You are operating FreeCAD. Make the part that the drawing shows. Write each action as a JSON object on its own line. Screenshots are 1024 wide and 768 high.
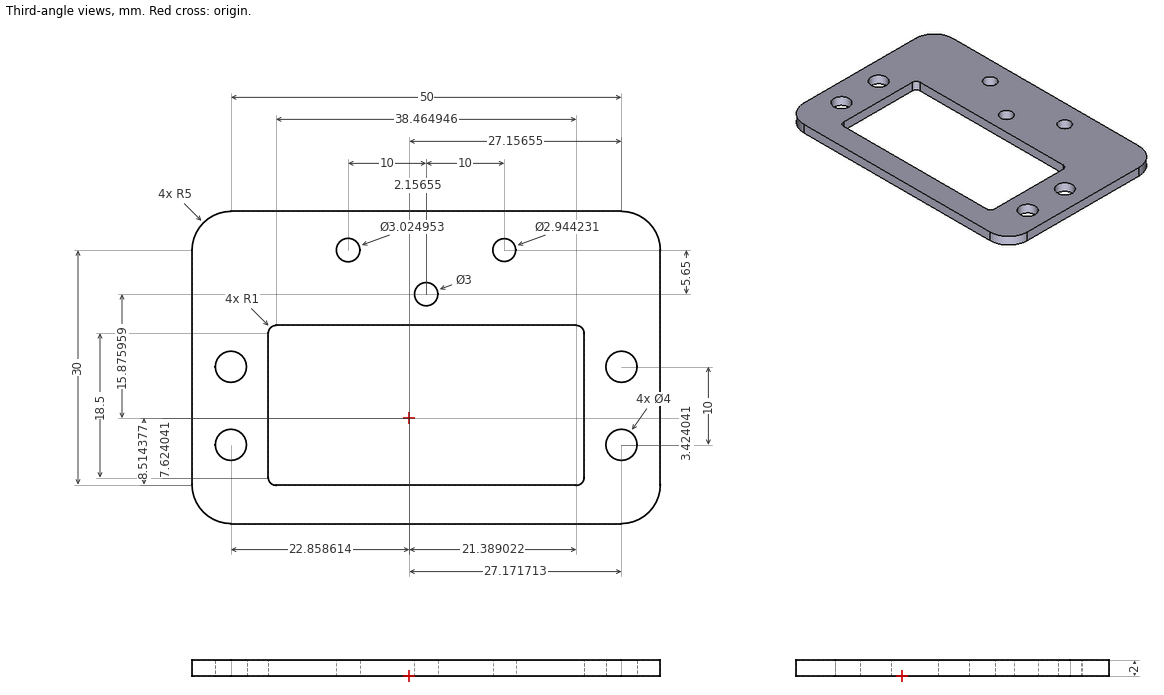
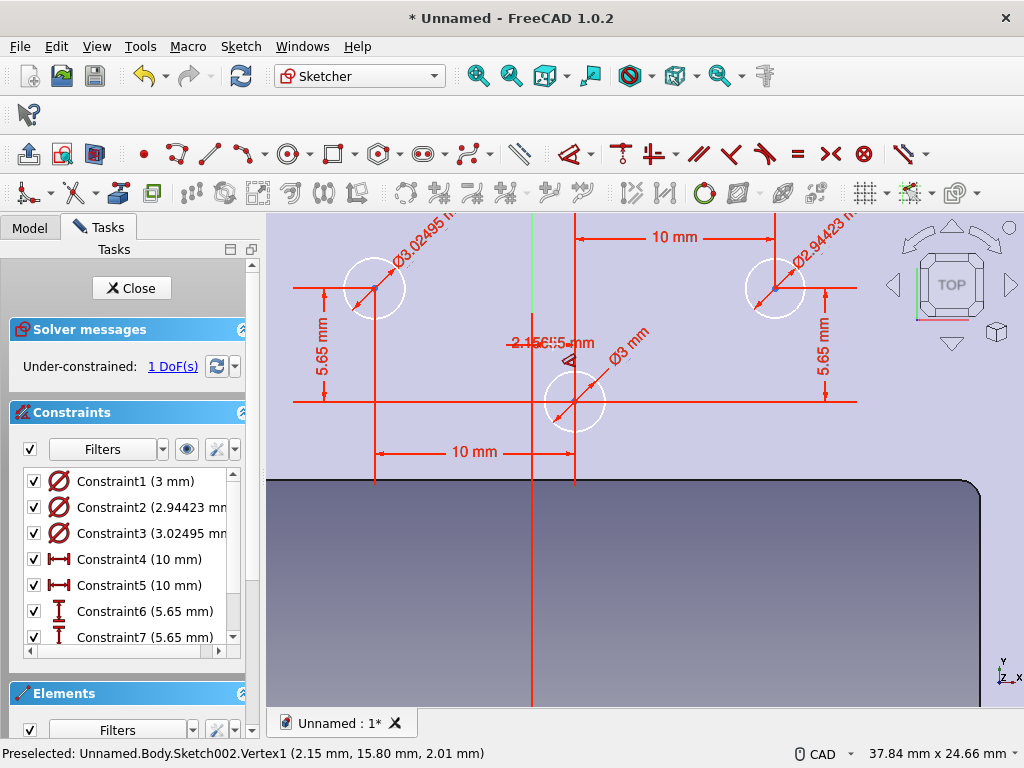
{"action": "left_click", "coordinate": [575, 402]}
{"action": "left_click", "coordinate": [498, 540]}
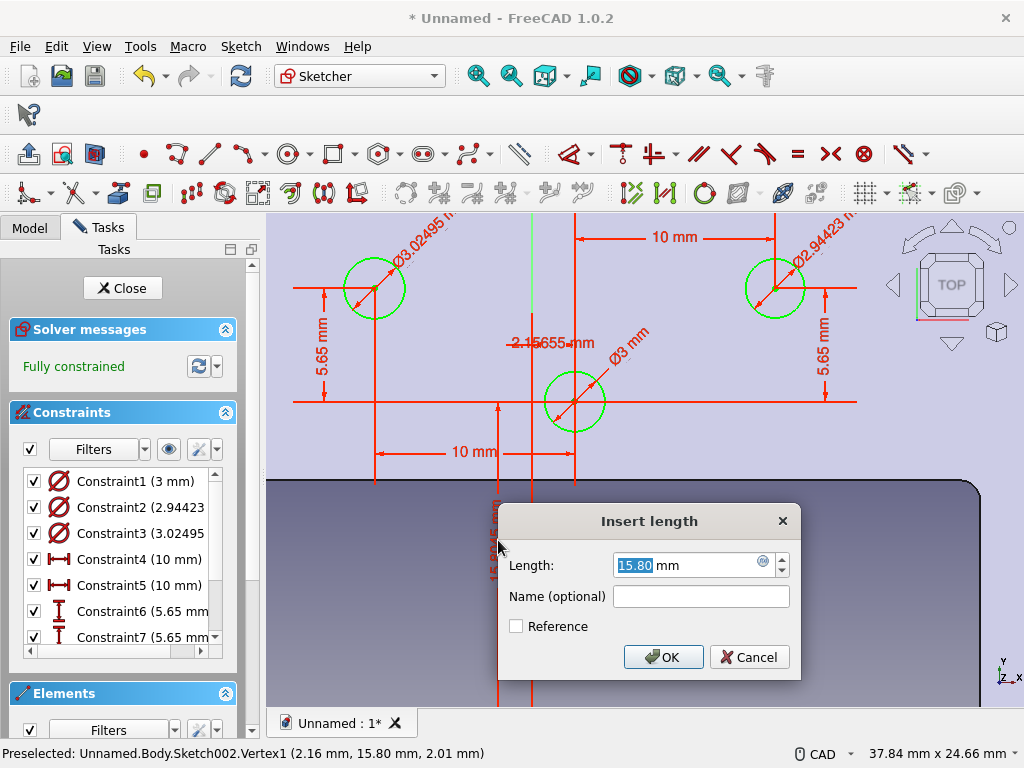
{"action": "type", "text": "15.875959"}
{"action": "key", "text": "Return"}
{"action": "key", "text": "Escape"}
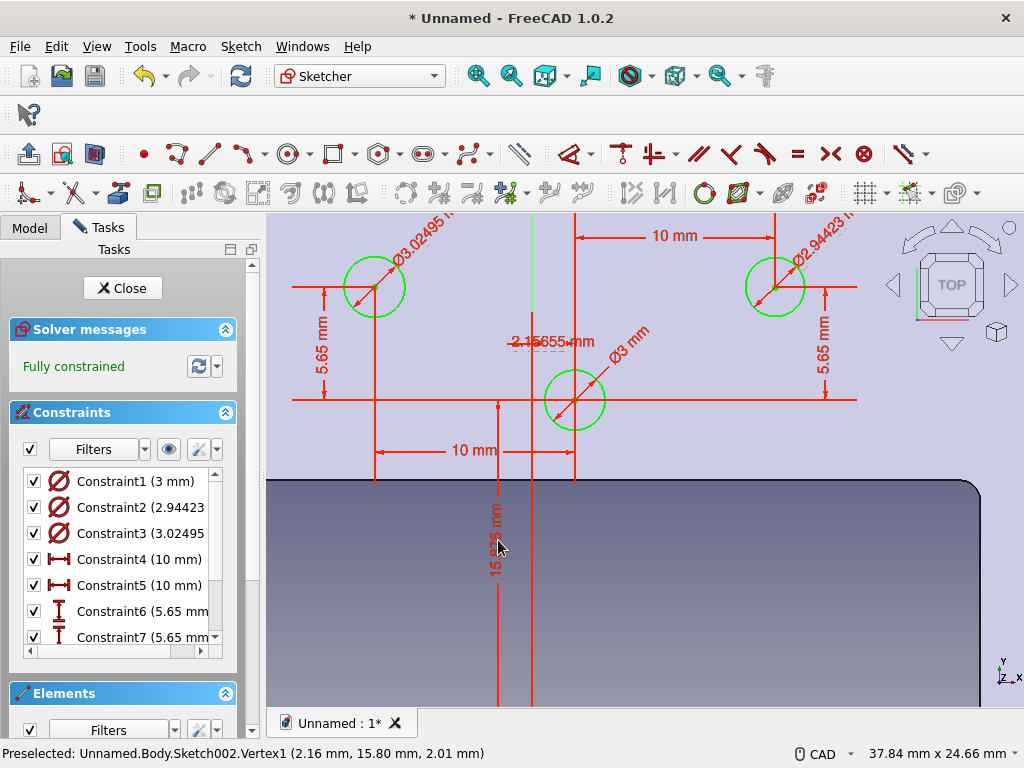
{"action": "left_click", "coordinate": [123, 288]}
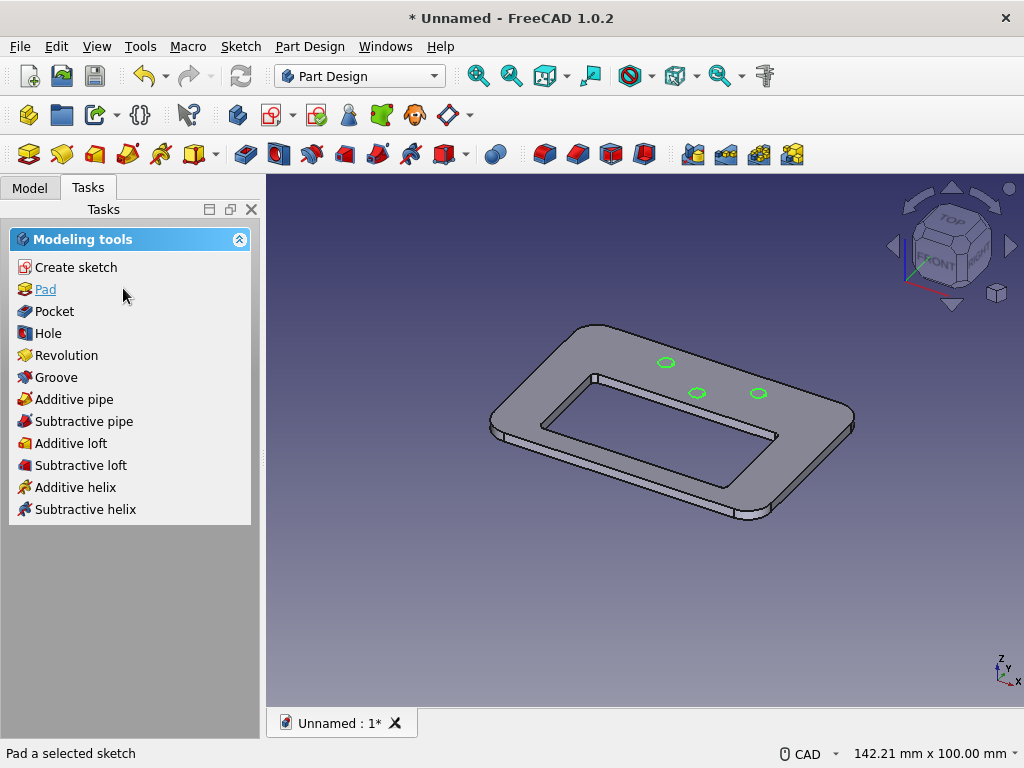
{"action": "left_click", "coordinate": [246, 154]}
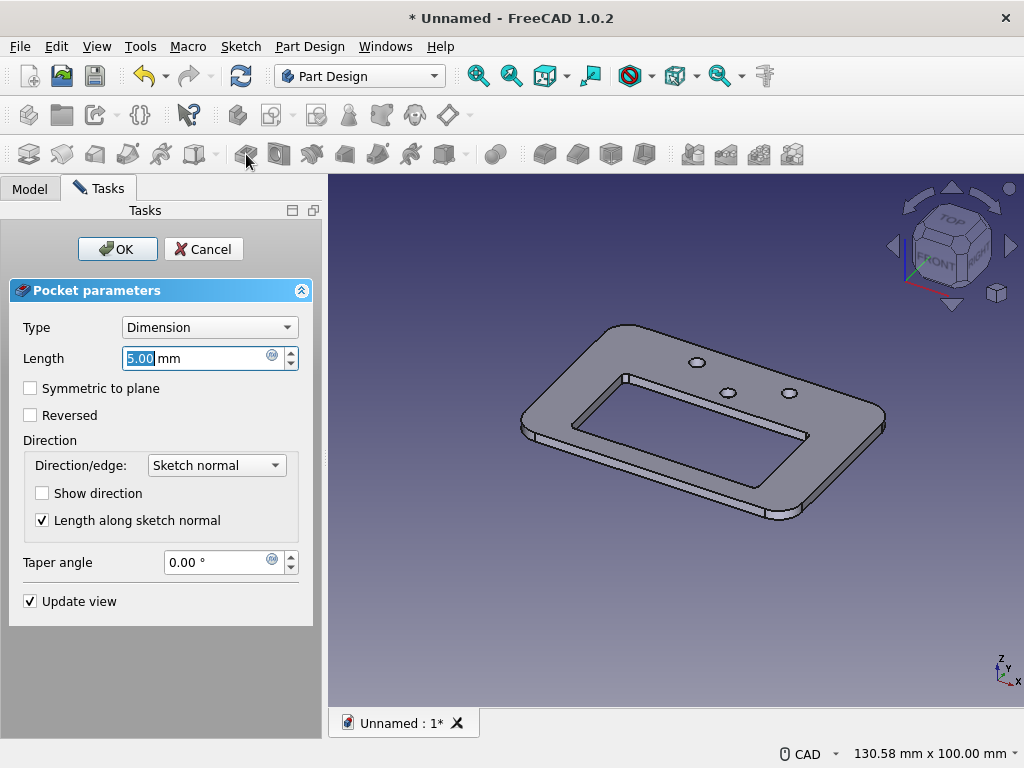
{"action": "left_click", "coordinate": [210, 328]}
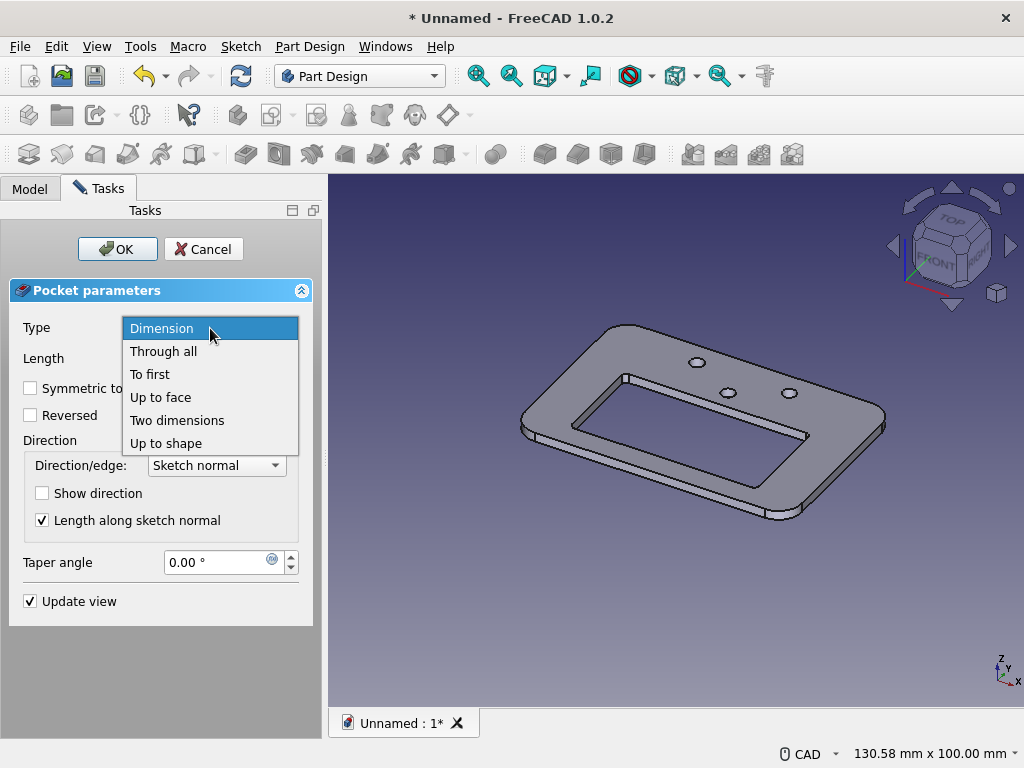
{"action": "left_click", "coordinate": [208, 352]}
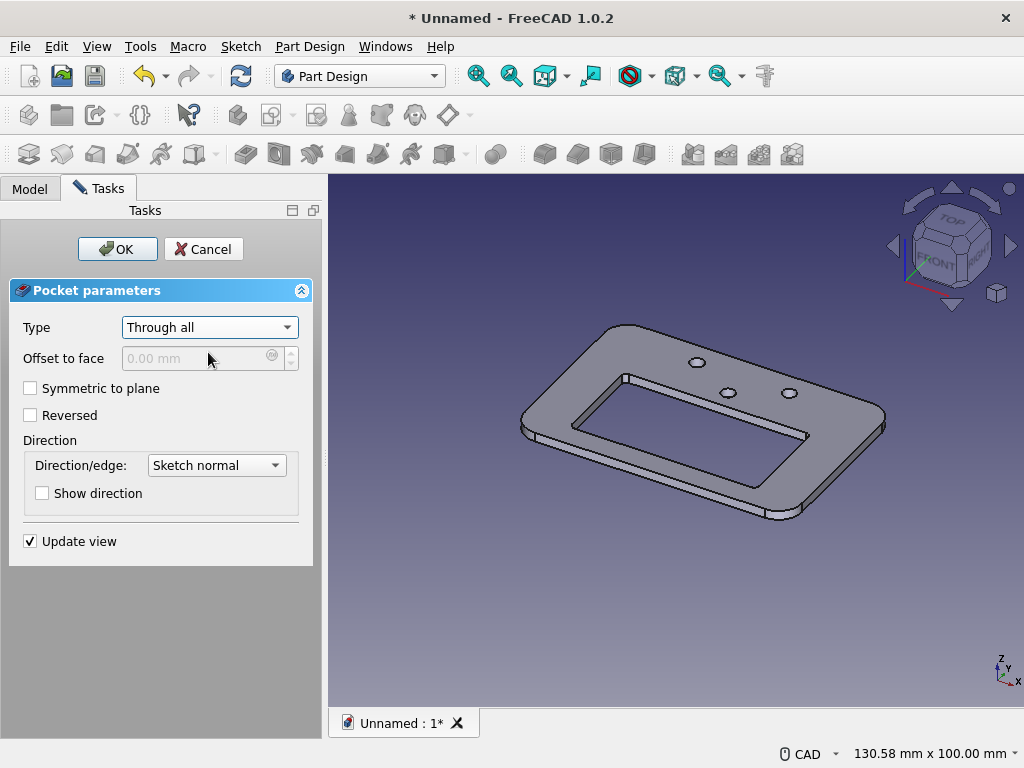
{"action": "left_click", "coordinate": [118, 249]}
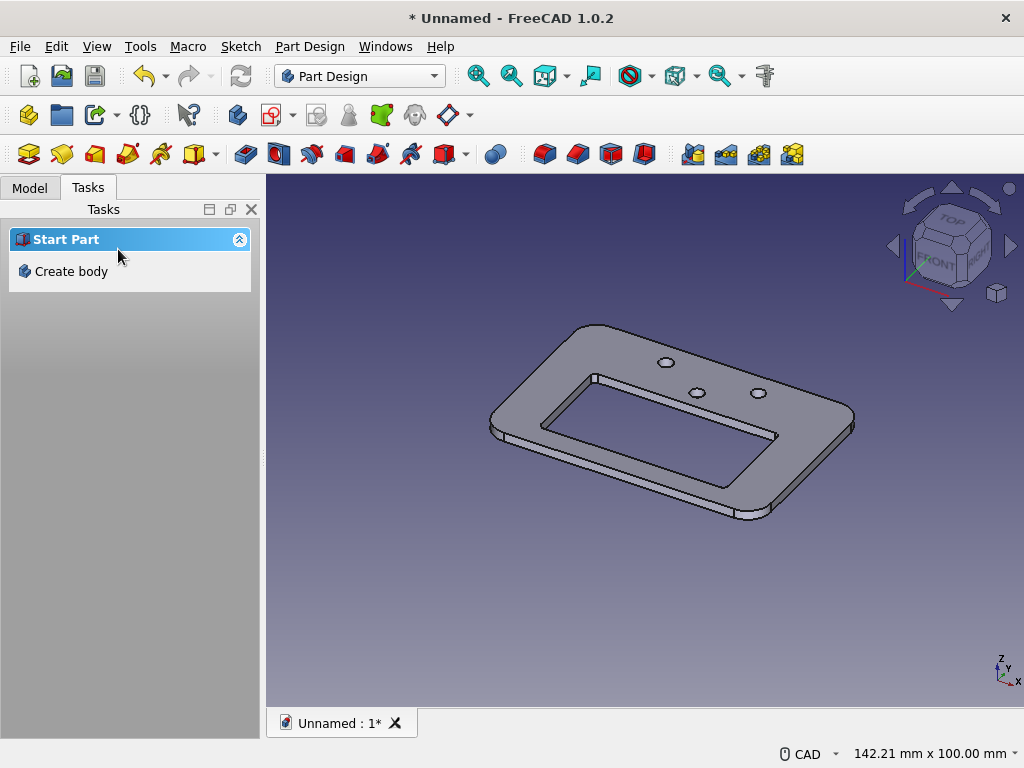
{"action": "left_click", "coordinate": [782, 413]}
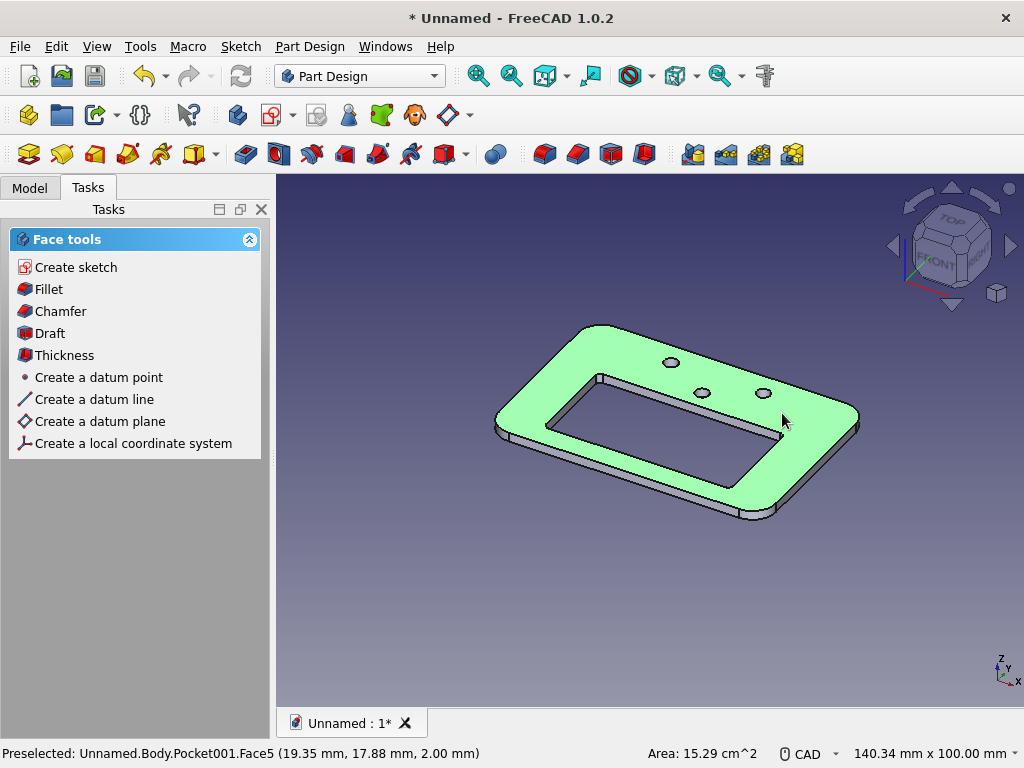
{"action": "left_click", "coordinate": [270, 116]}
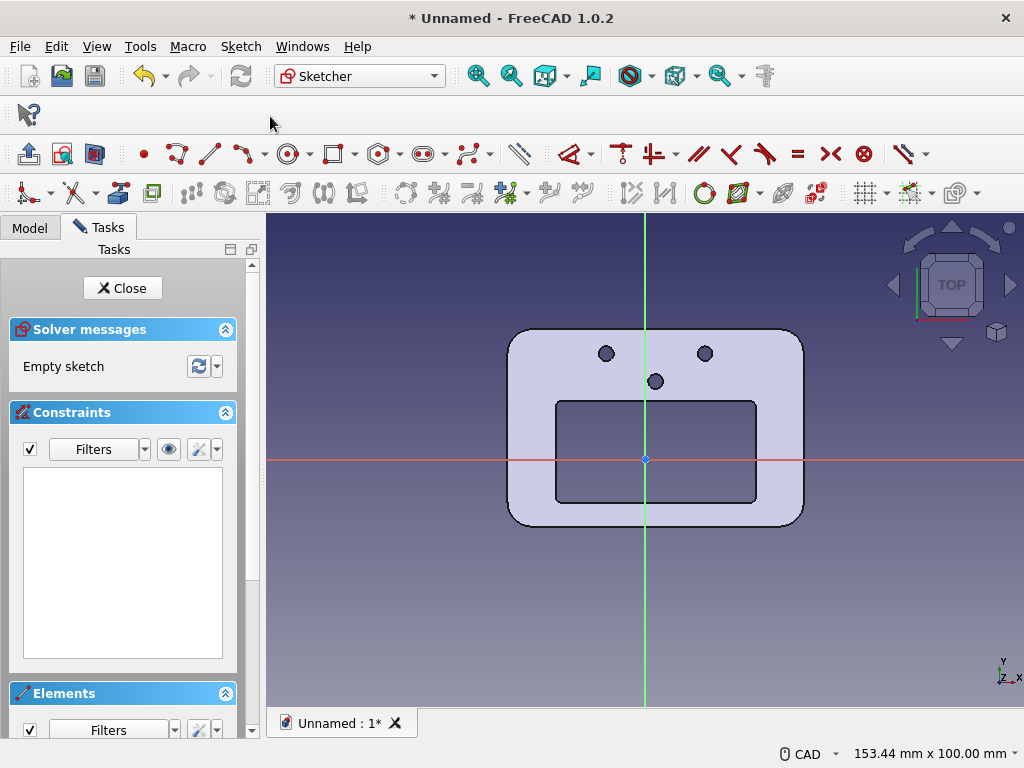
{"action": "scroll", "coordinate": [817, 436], "scroll_direction": "up", "scroll_amount": 2}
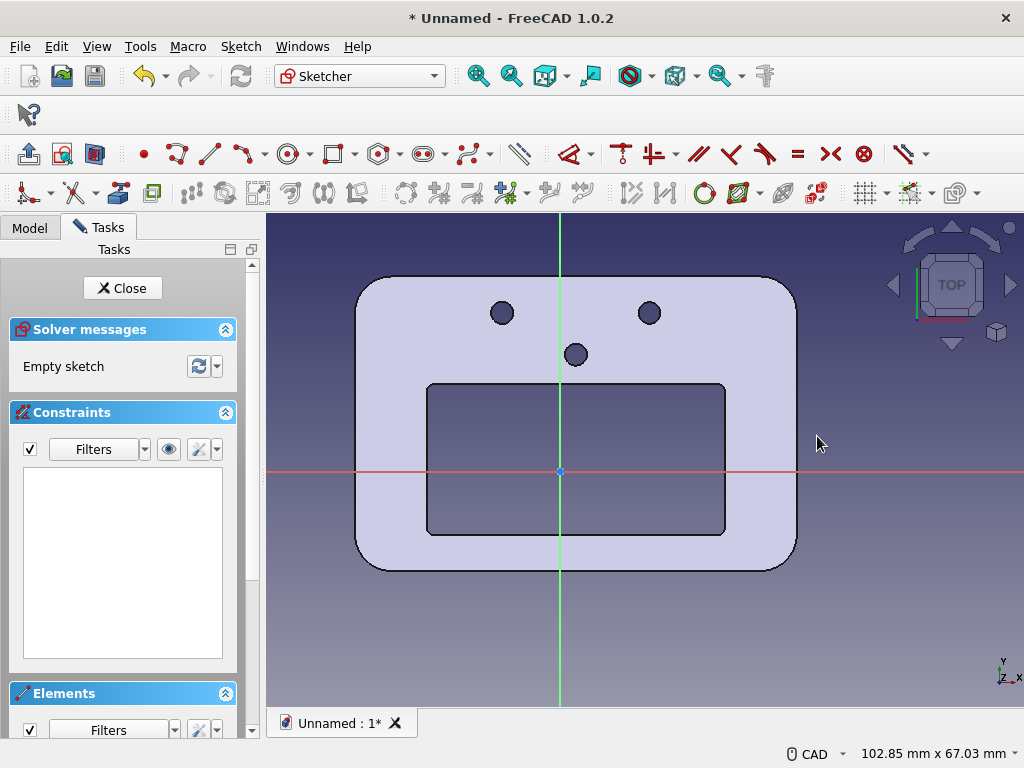
{"action": "left_click", "coordinate": [288, 154]}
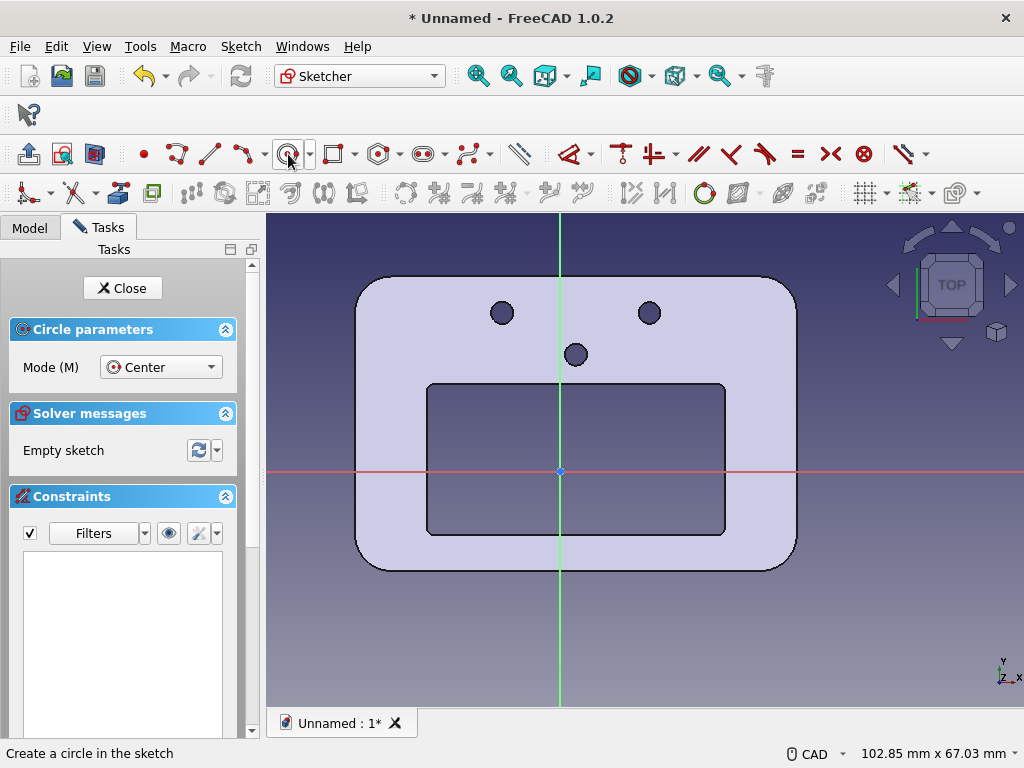
{"action": "scroll", "coordinate": [760, 497], "scroll_direction": "up", "scroll_amount": 3}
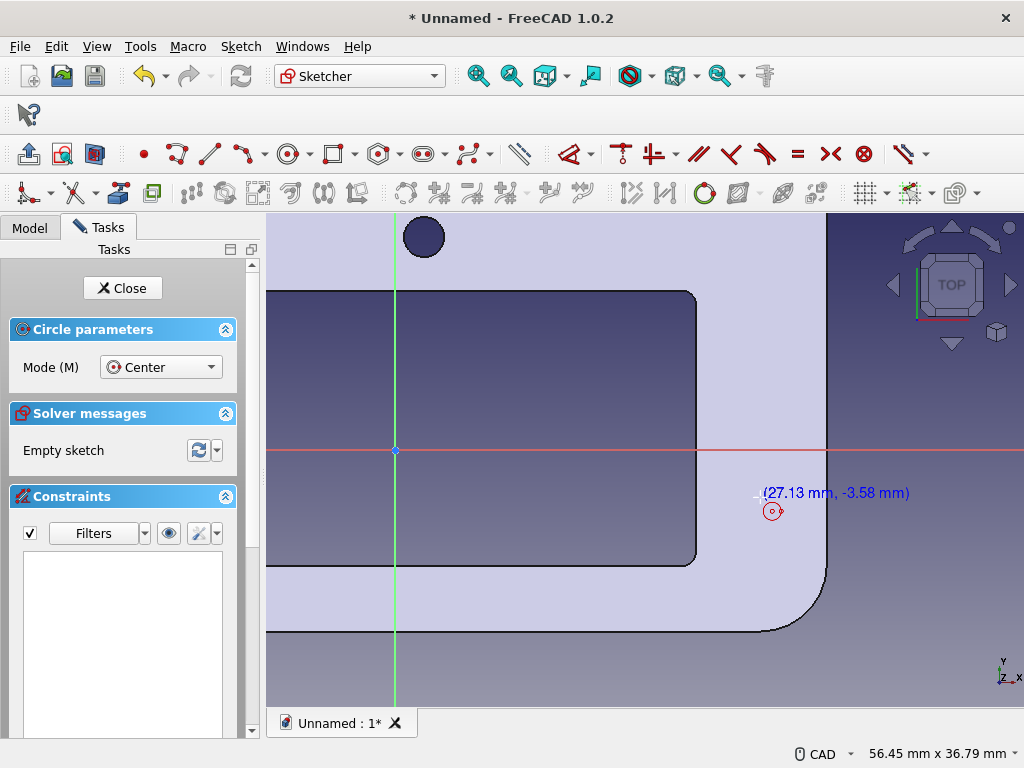
{"action": "left_click", "coordinate": [760, 496]}
{"action": "left_click", "coordinate": [779, 477]}